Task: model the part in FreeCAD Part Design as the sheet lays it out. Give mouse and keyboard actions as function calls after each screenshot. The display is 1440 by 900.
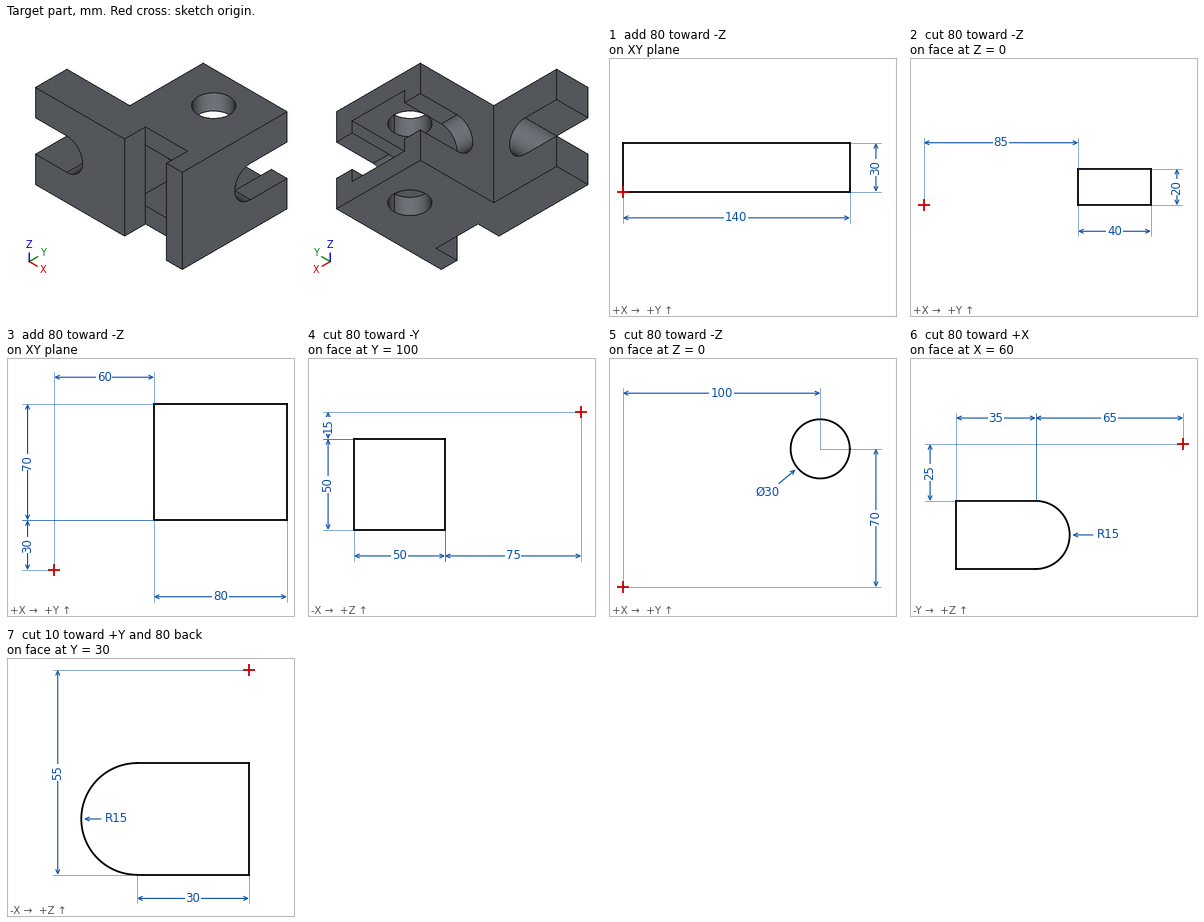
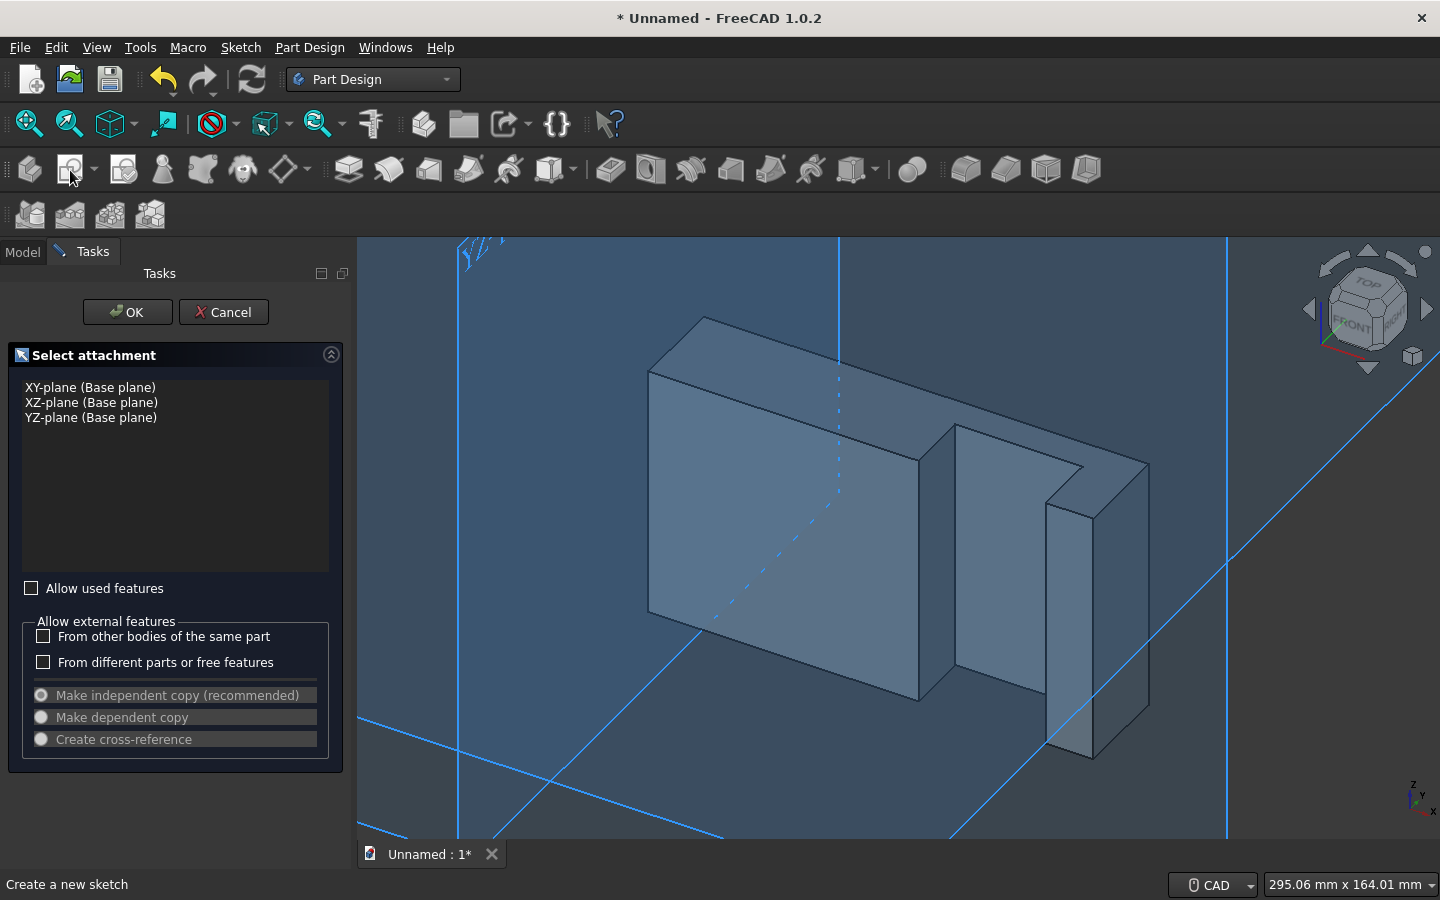
click(82, 388)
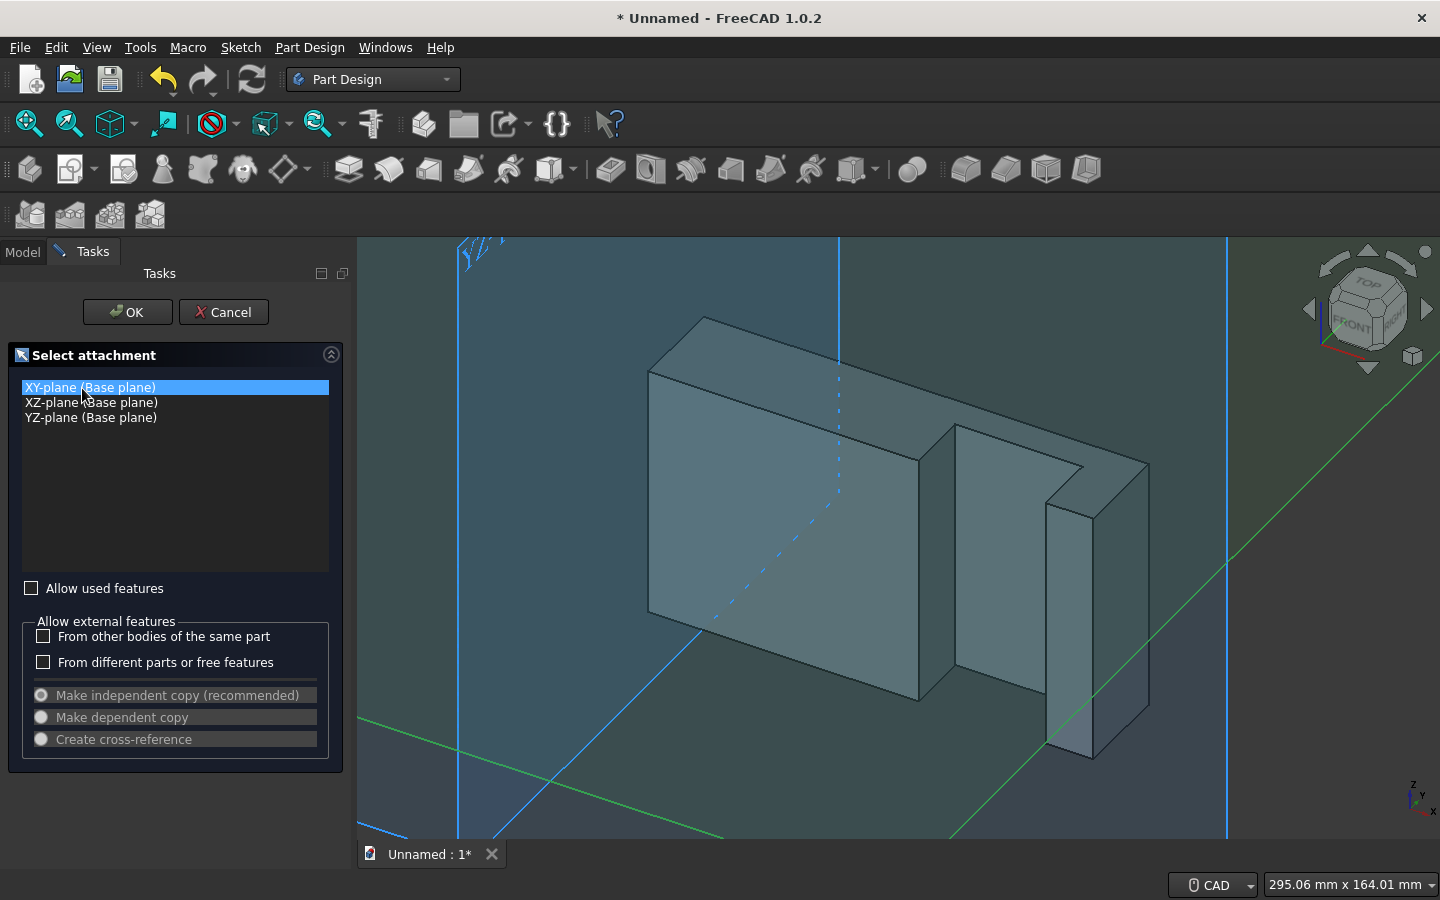
click(128, 312)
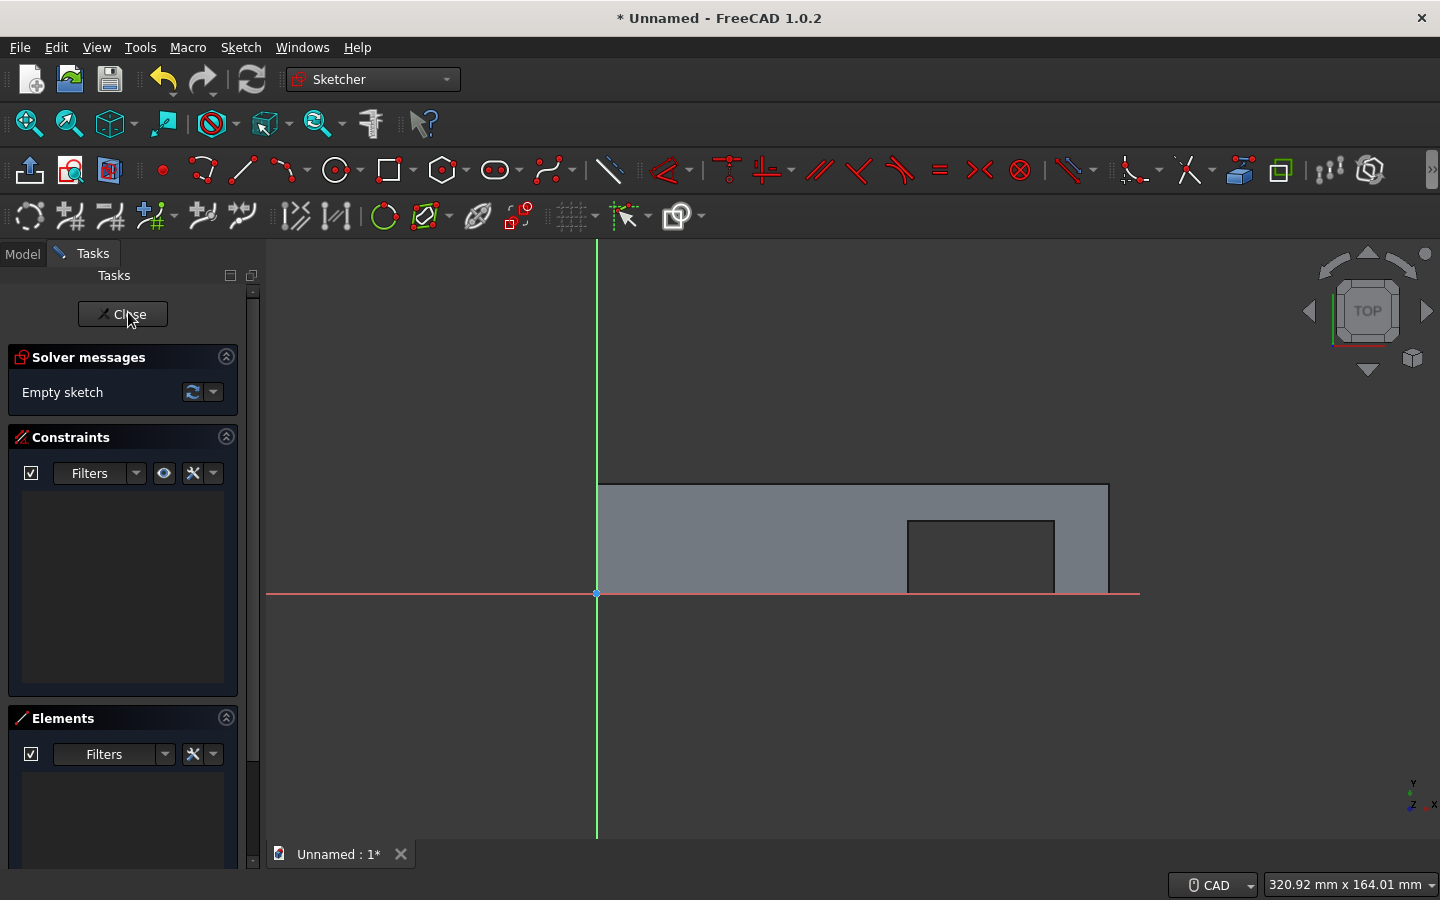
scroll(475, 811, down, 1)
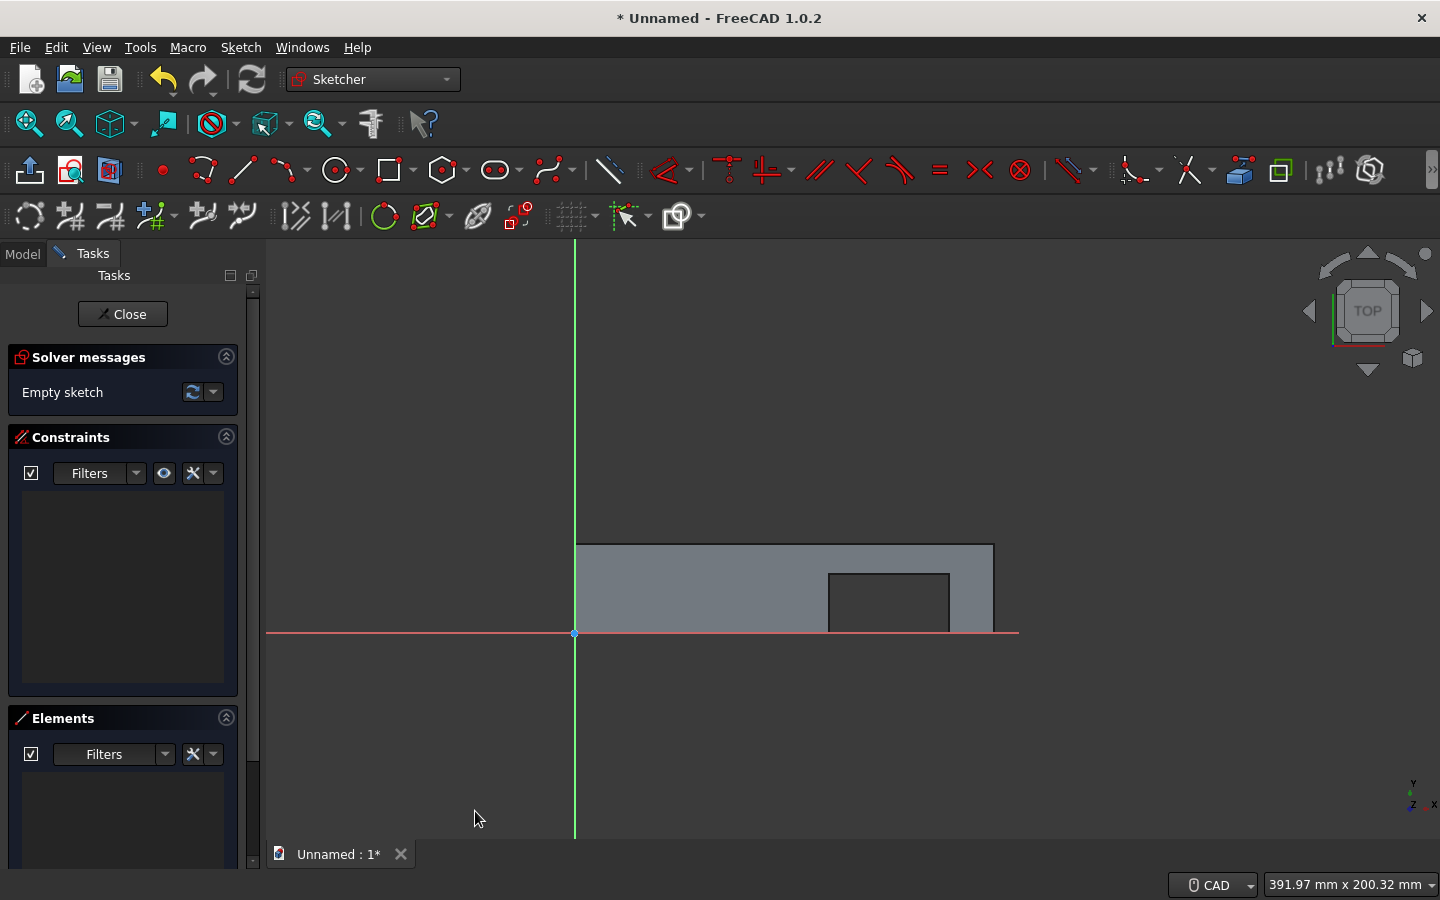
key(g)
key(r)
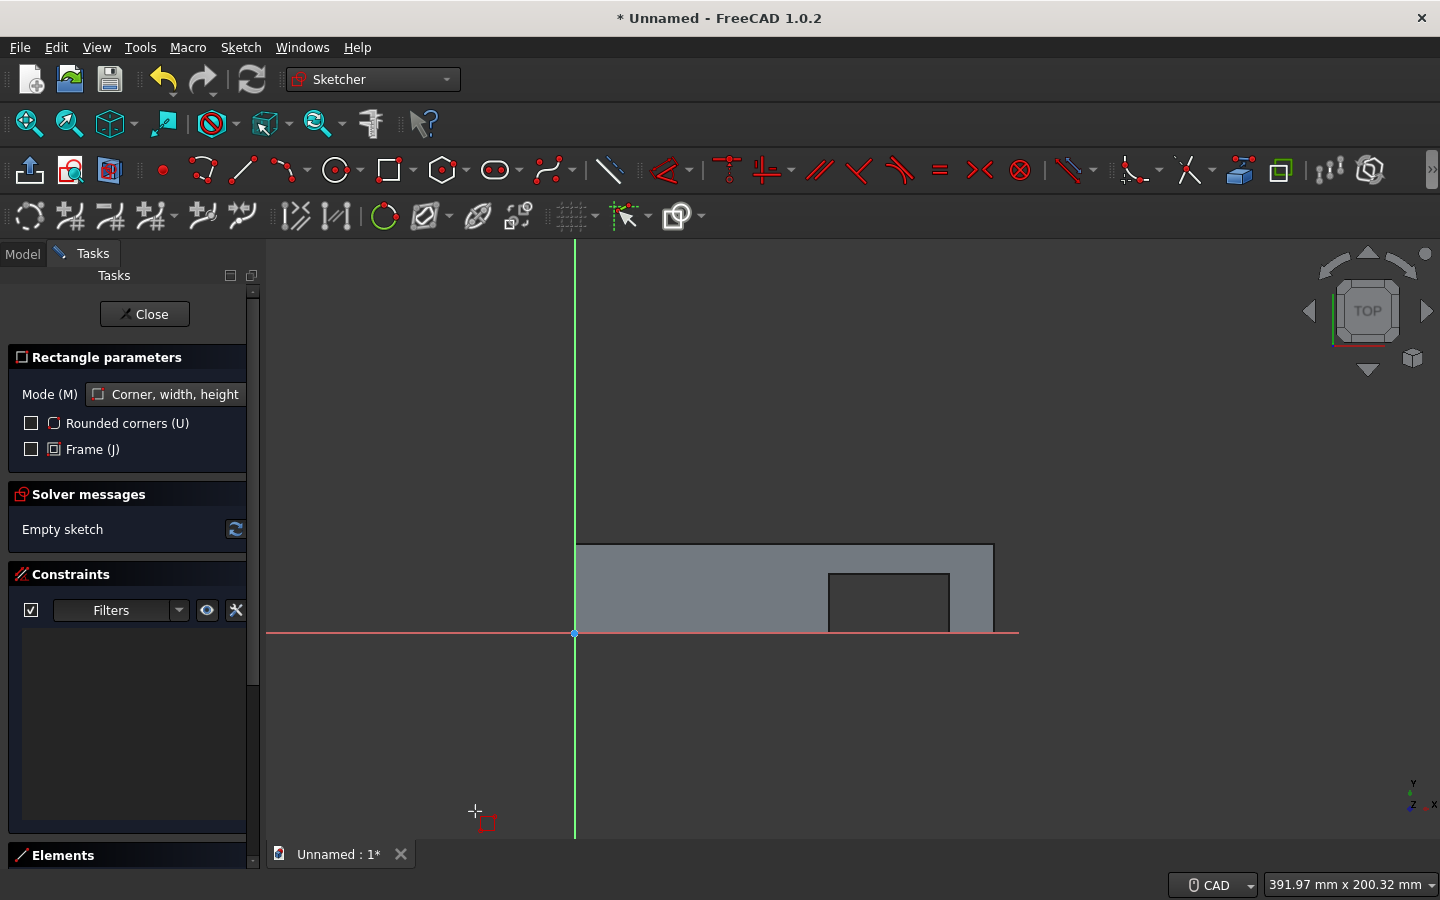
click(755, 334)
click(994, 544)
key(Escape)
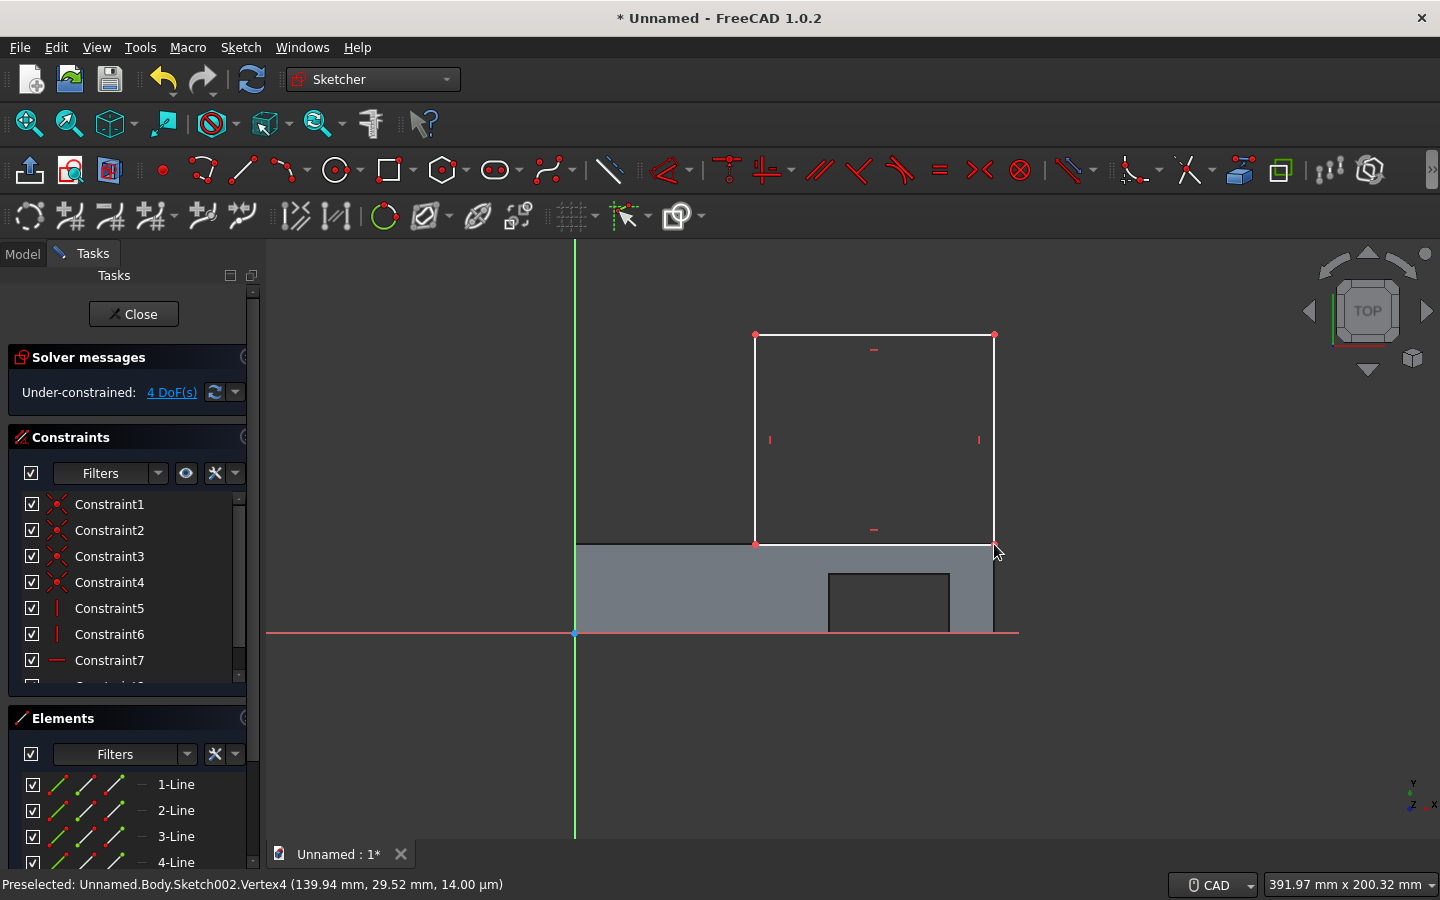
key(d)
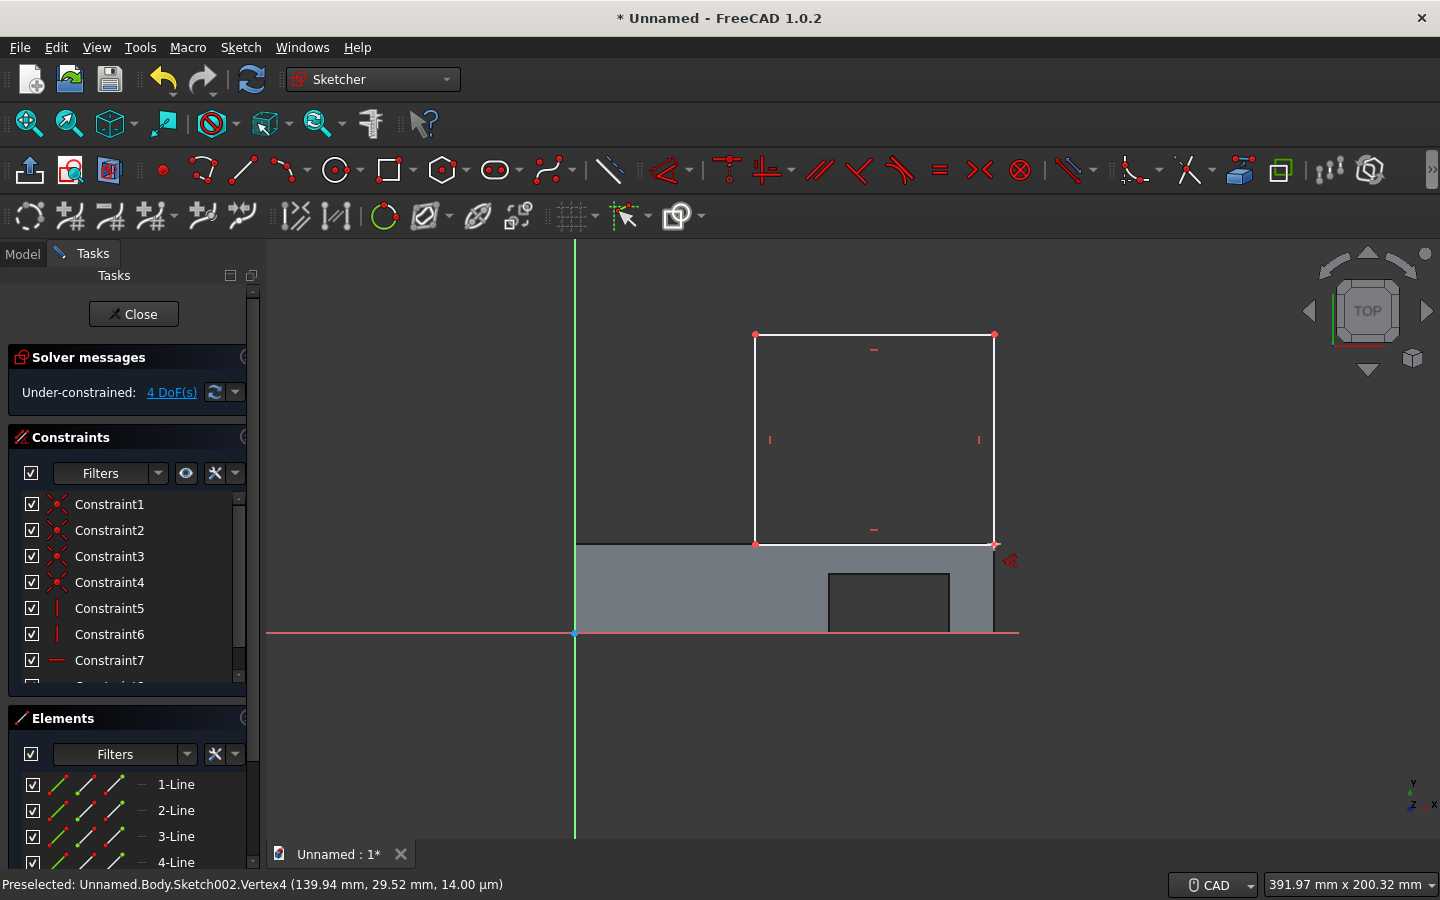
click(755, 398)
click(721, 440)